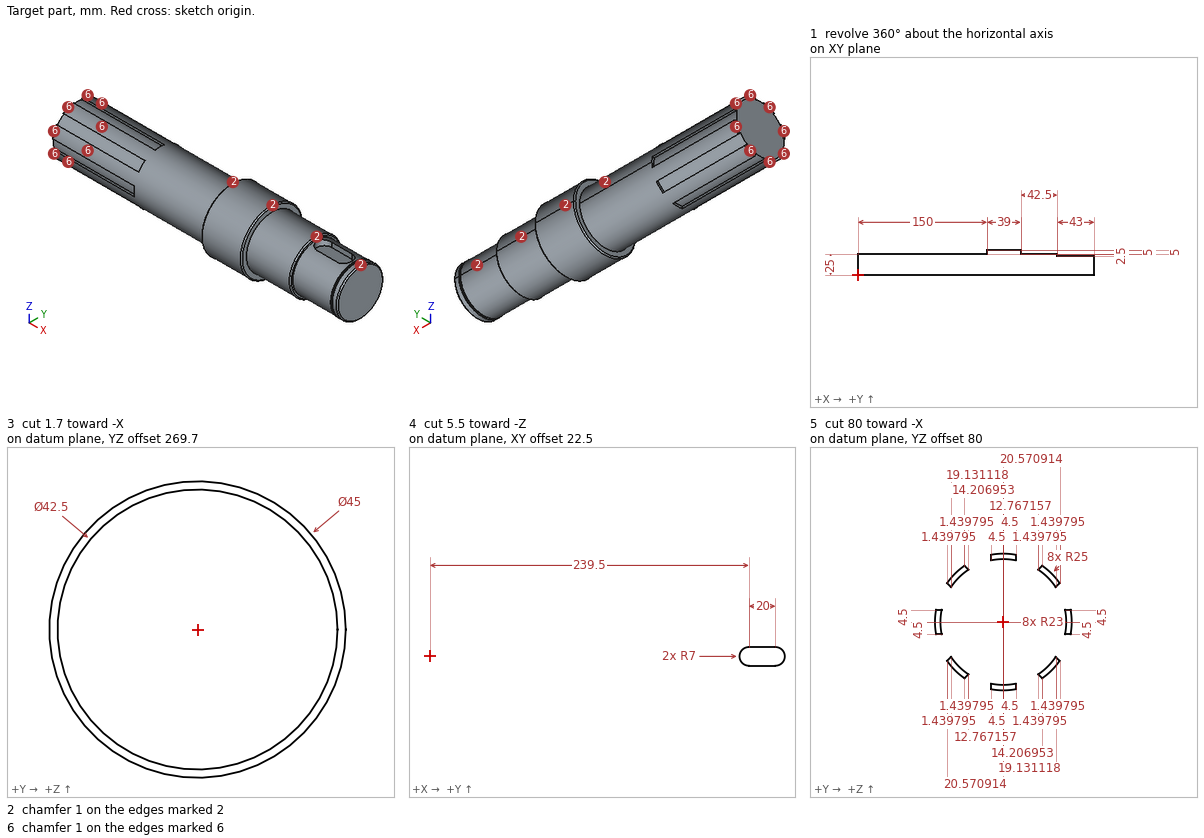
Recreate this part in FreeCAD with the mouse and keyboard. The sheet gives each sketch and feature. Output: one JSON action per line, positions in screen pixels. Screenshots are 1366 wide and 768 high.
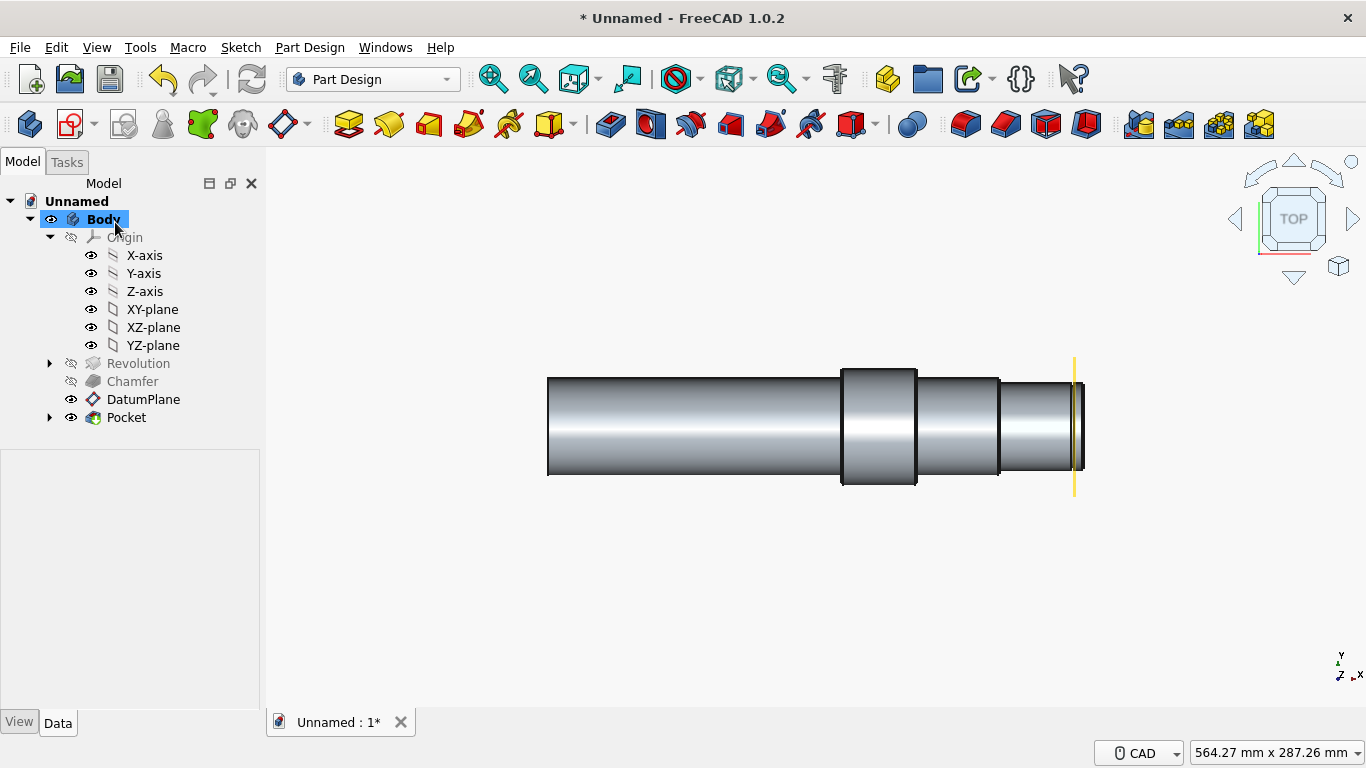
{"action": "left_click", "coordinate": [116, 399]}
{"action": "key", "text": "space"}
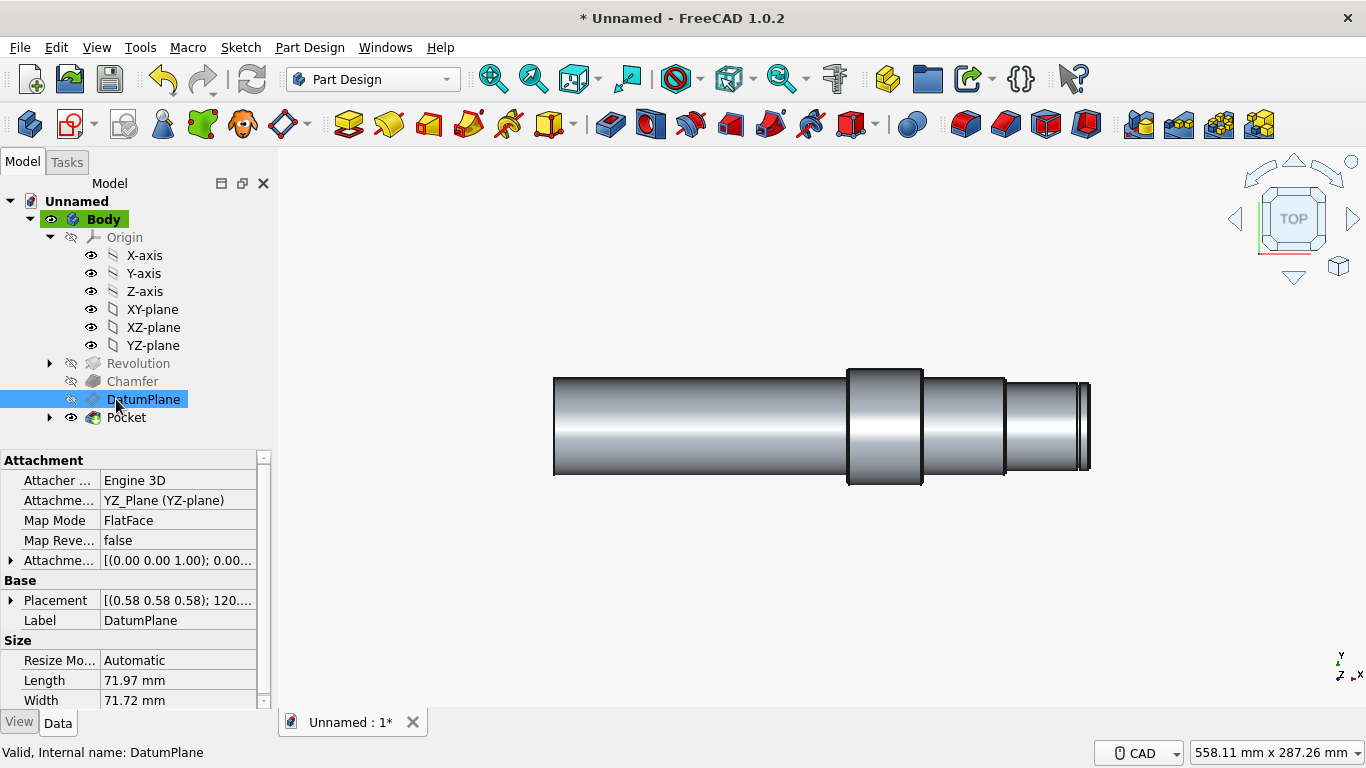
{"action": "left_click", "coordinate": [136, 309]}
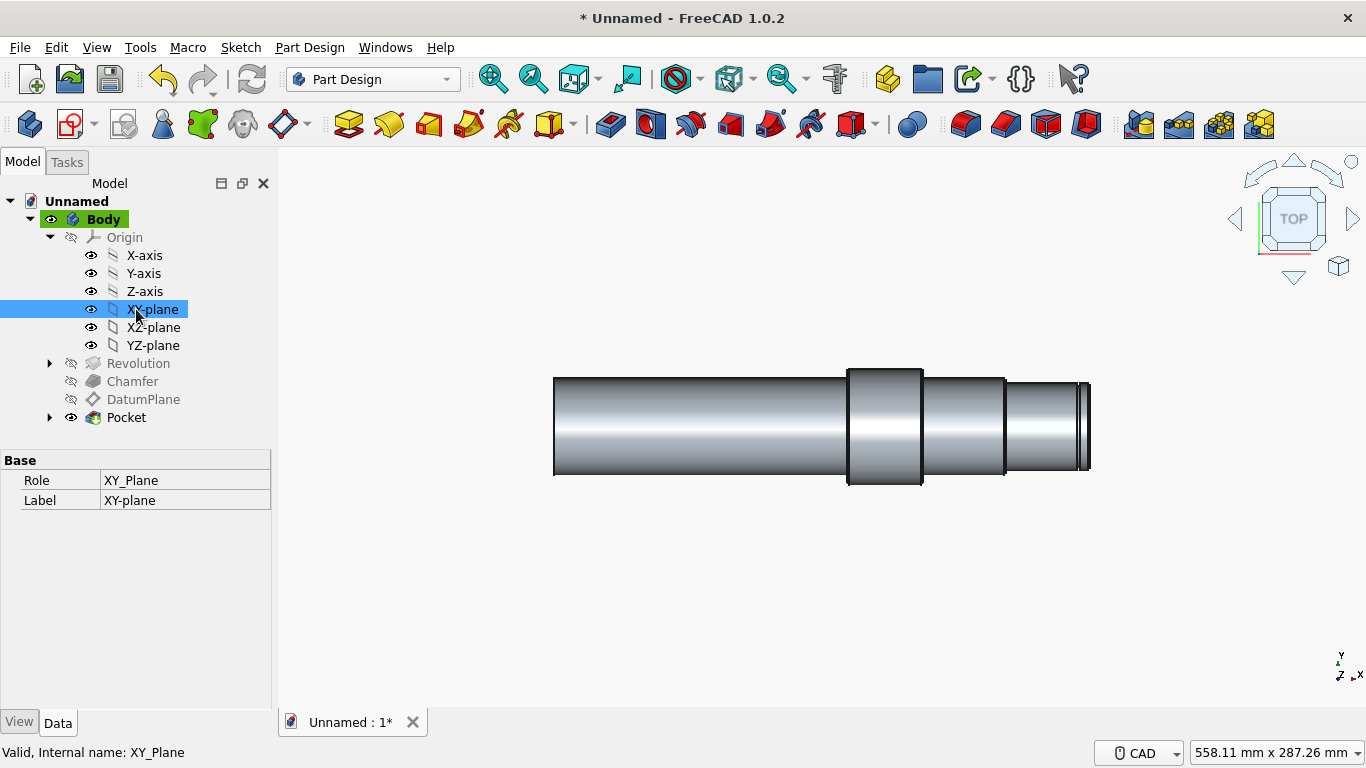
{"action": "left_click", "coordinate": [284, 124]}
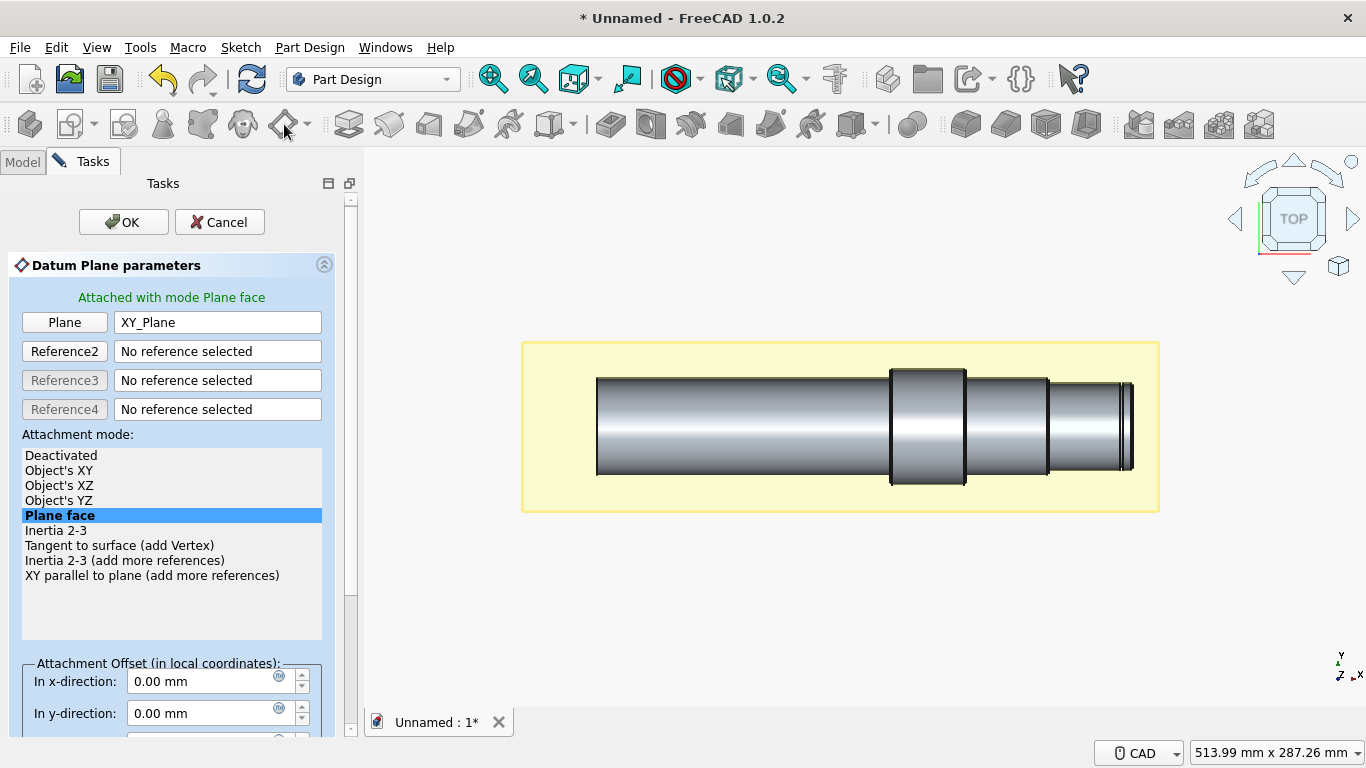
{"action": "scroll", "coordinate": [351, 464], "scroll_direction": "down", "scroll_amount": 2}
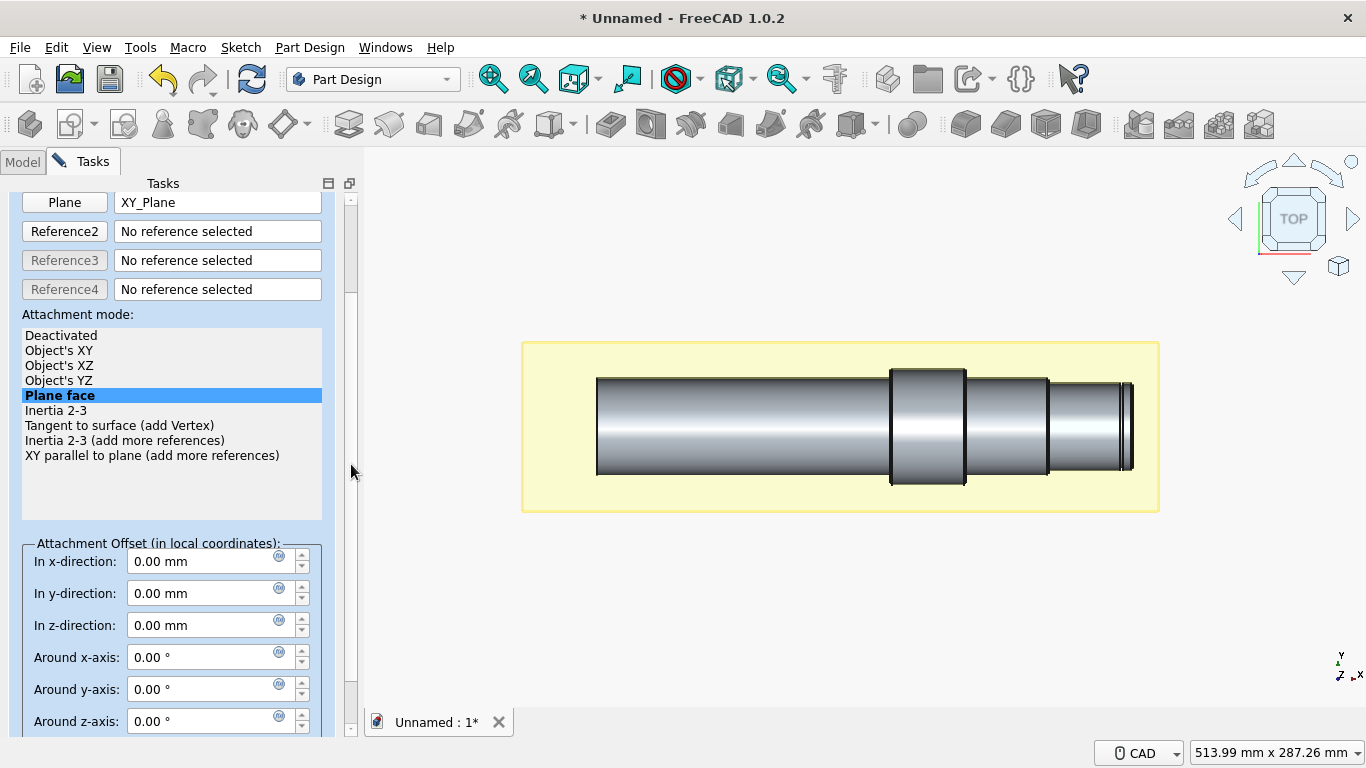
{"action": "triple_click", "coordinate": [210, 625]}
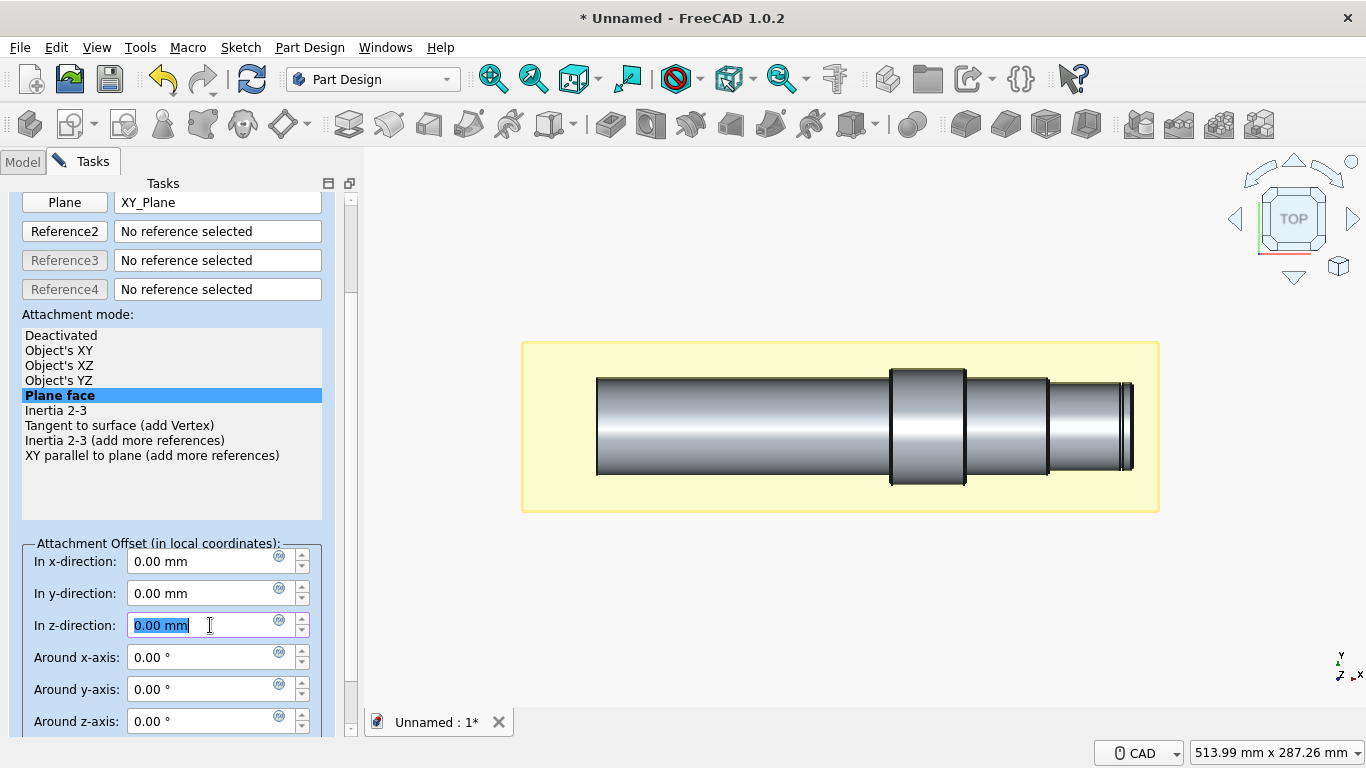
{"action": "type", "text": "22.5"}
{"action": "key", "text": "Tab"}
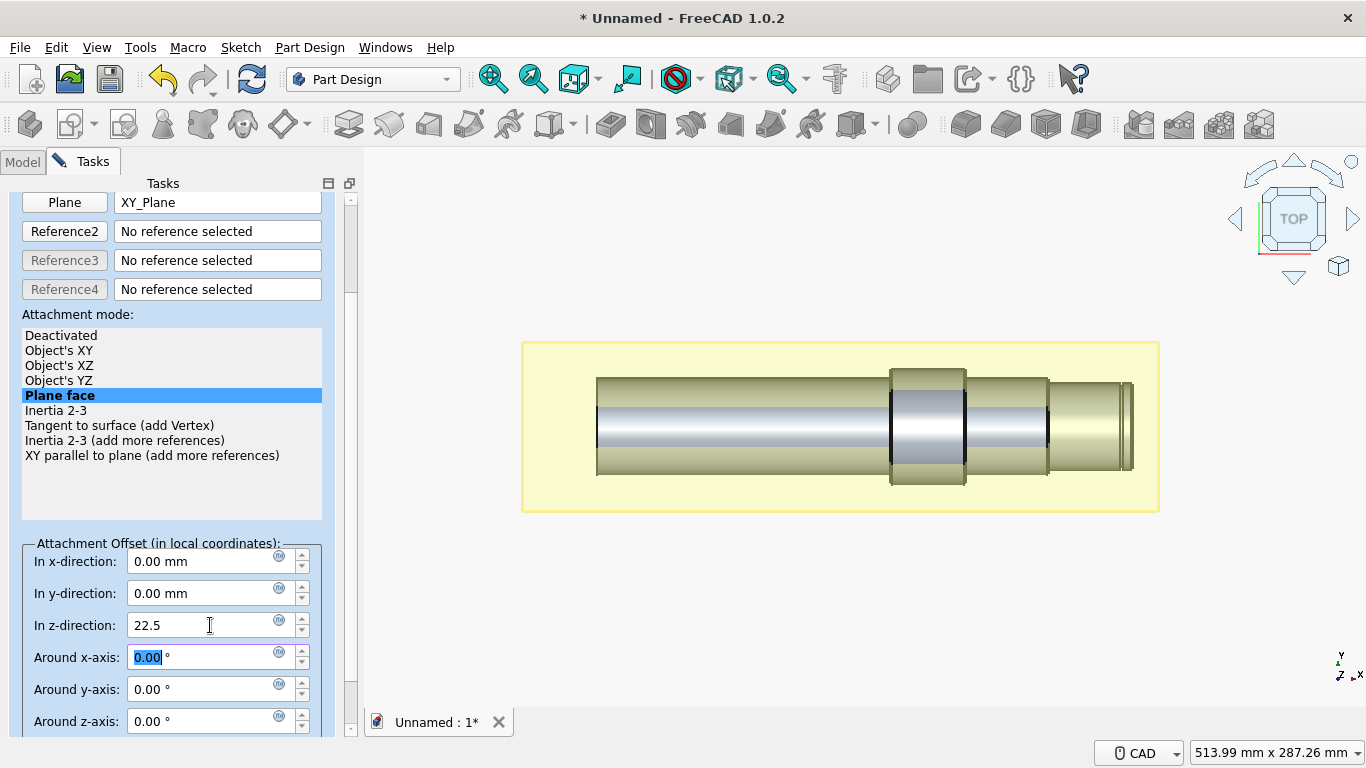
{"action": "scroll", "coordinate": [351, 464], "scroll_direction": "up", "scroll_amount": 3}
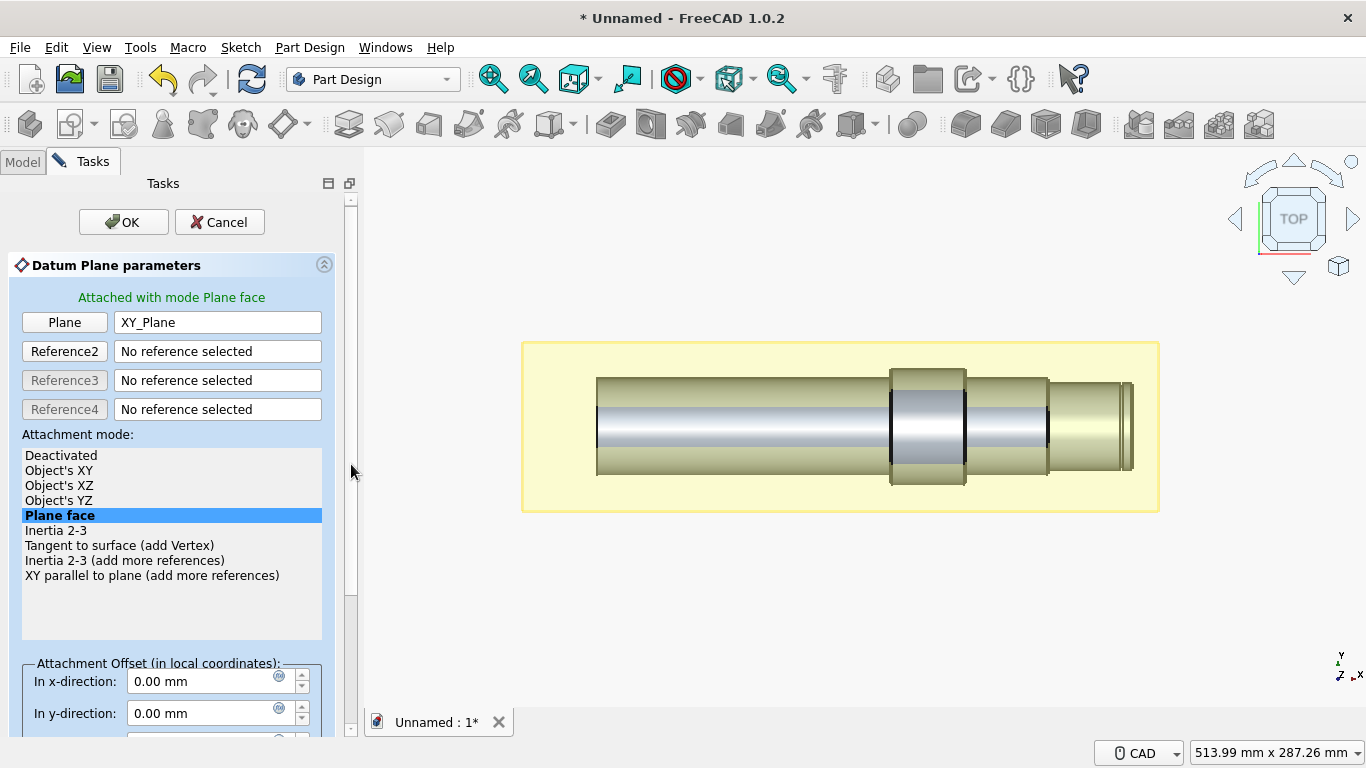
{"action": "left_click", "coordinate": [124, 222]}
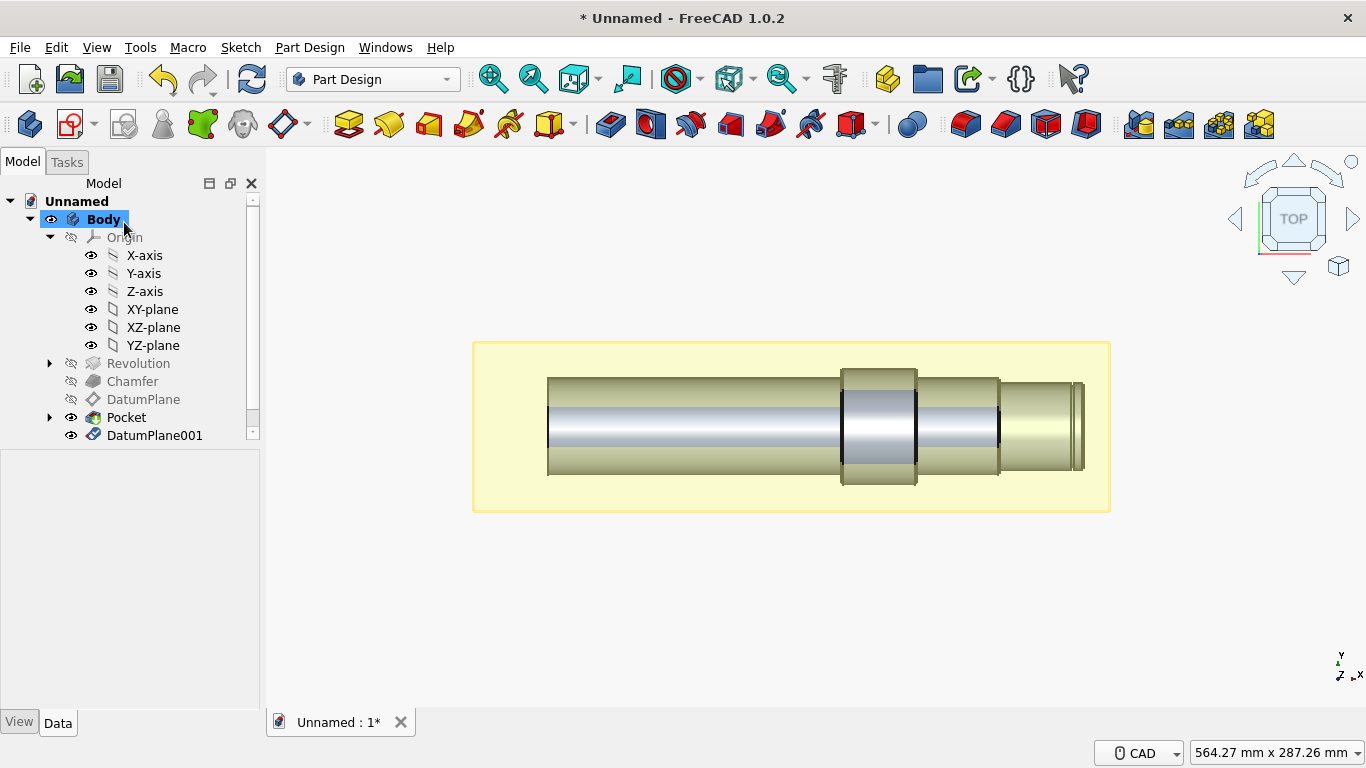
{"action": "left_click", "coordinate": [116, 435]}